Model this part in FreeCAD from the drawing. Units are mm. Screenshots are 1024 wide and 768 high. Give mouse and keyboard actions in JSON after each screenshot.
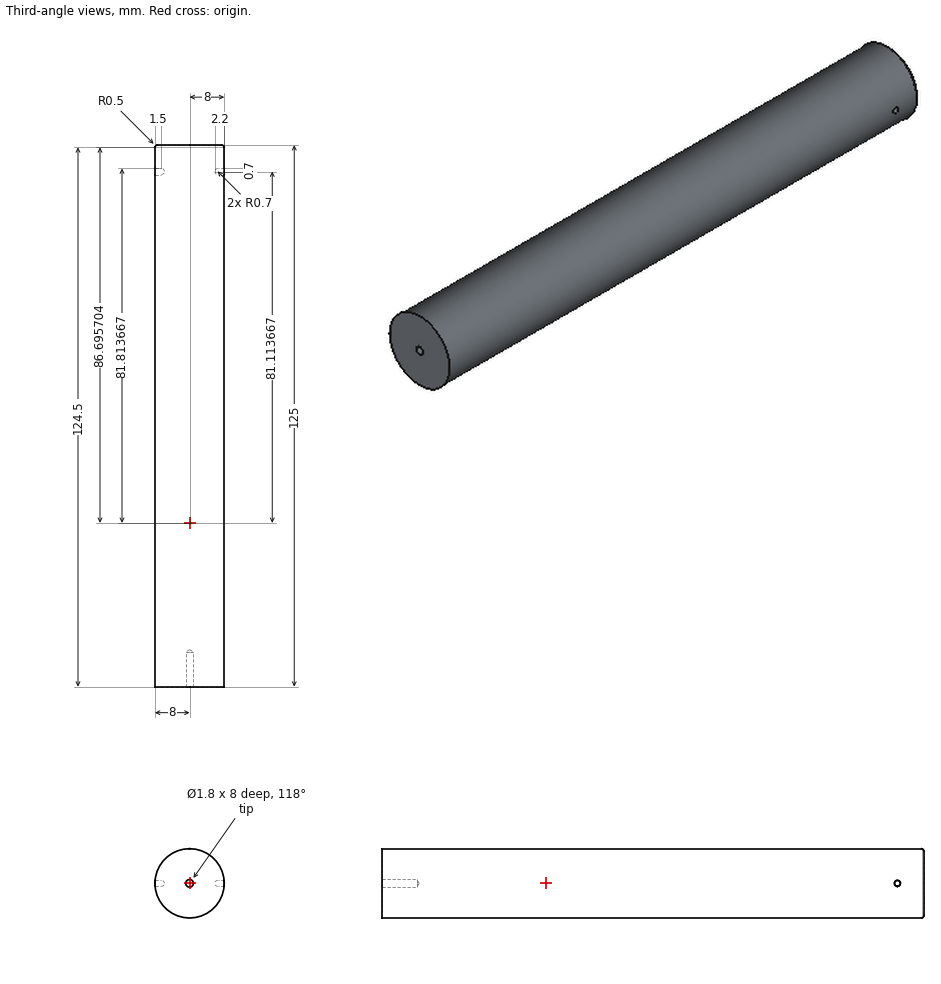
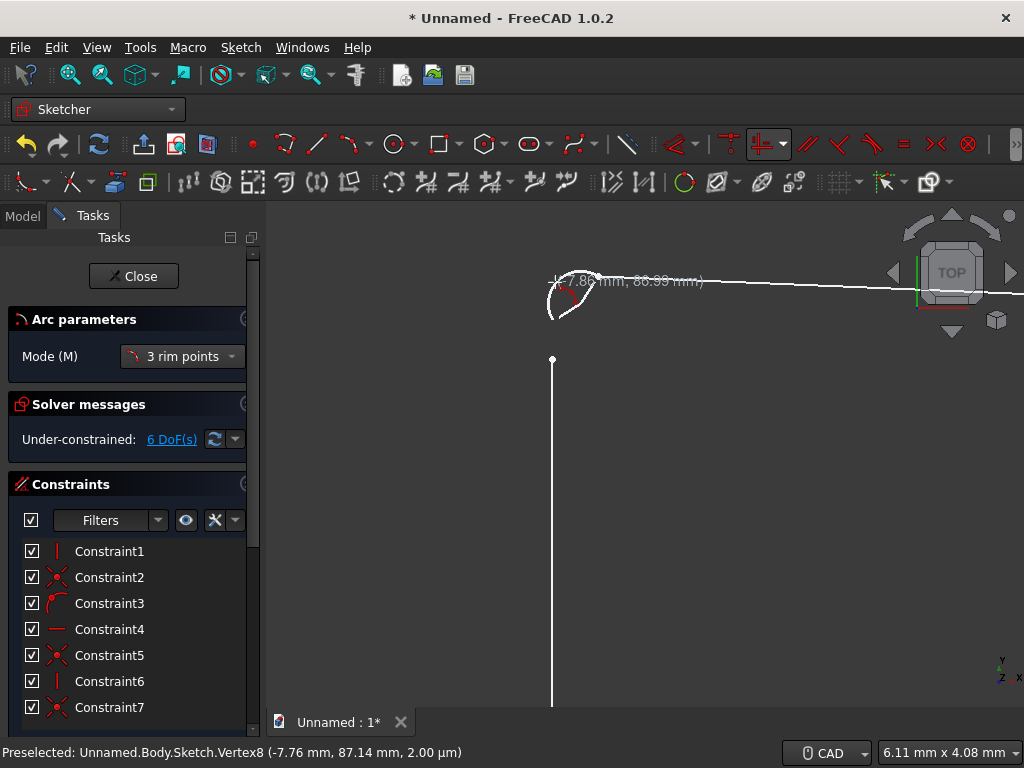
{"action": "left_click", "coordinate": [554, 279]}
{"action": "key", "text": "Escape"}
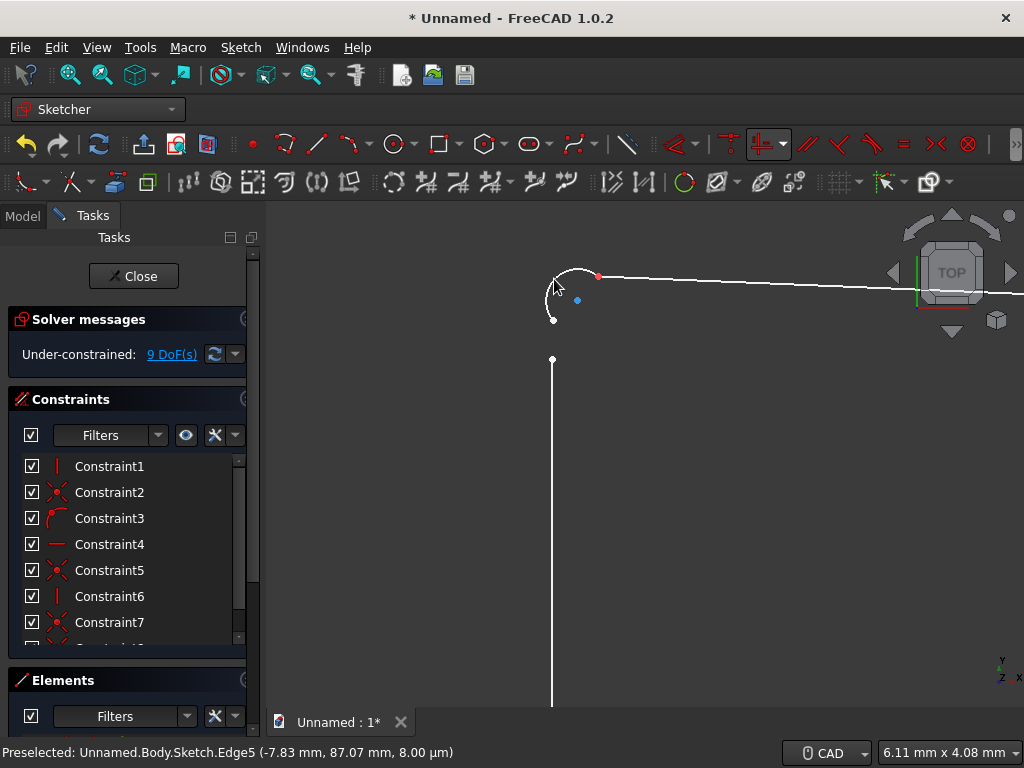
{"action": "scroll", "coordinate": [576, 454], "scroll_direction": "down", "scroll_amount": 15}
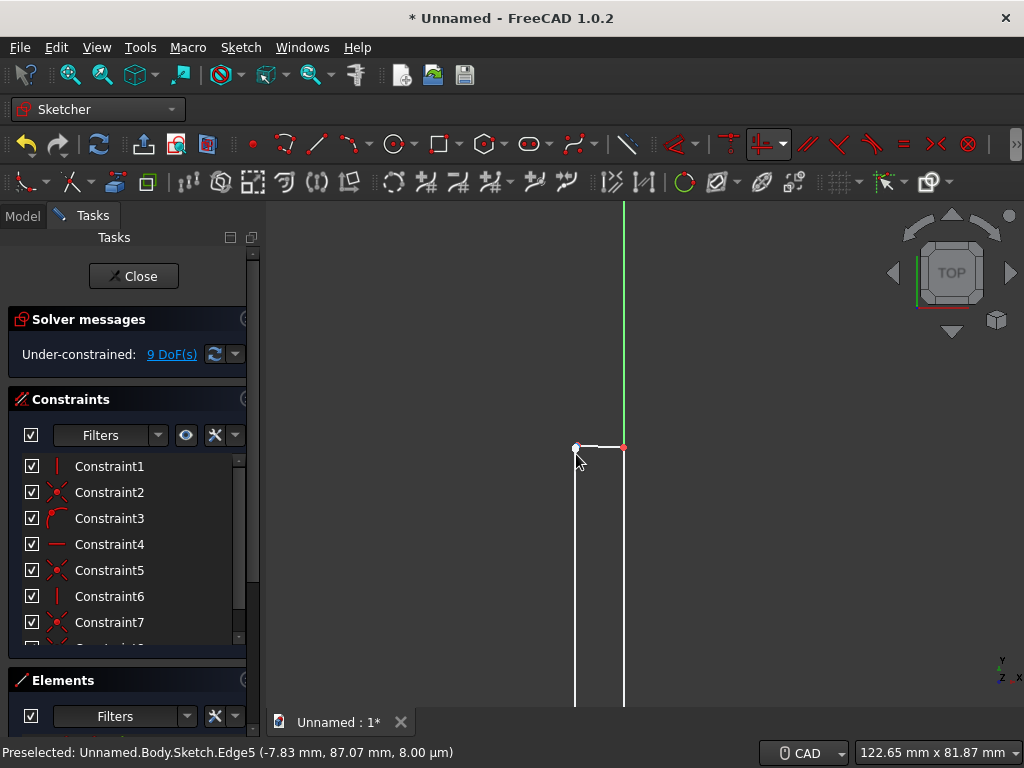
{"action": "scroll", "coordinate": [563, 235], "scroll_direction": "down", "scroll_amount": 5}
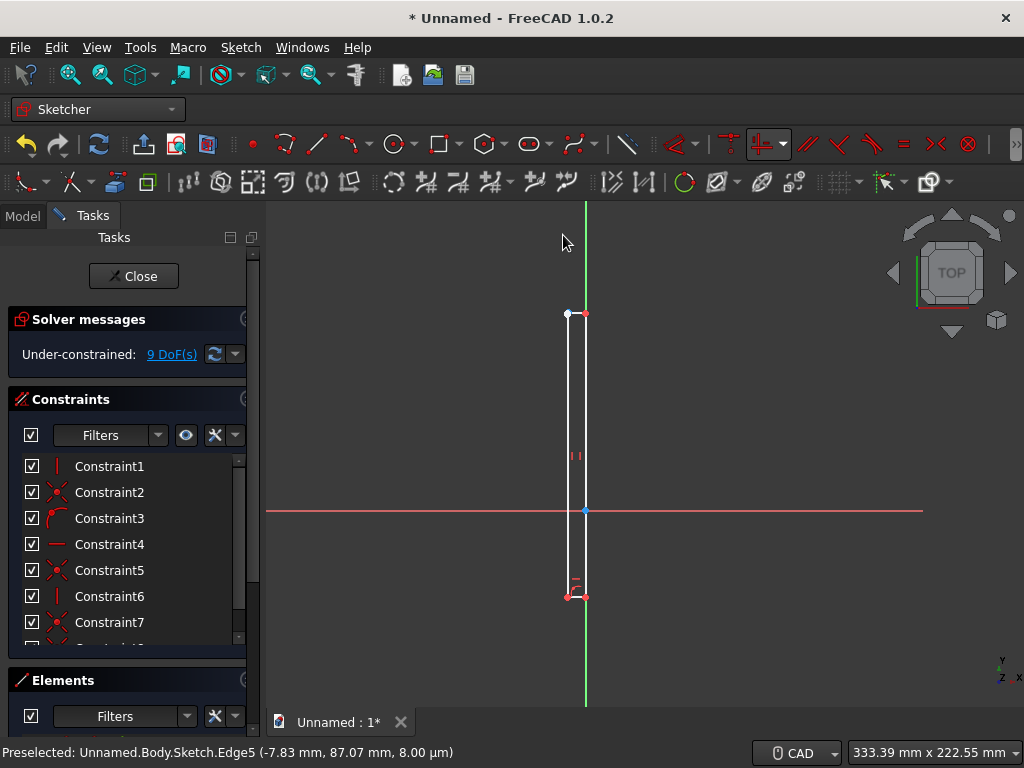
{"action": "left_click", "coordinate": [568, 399]}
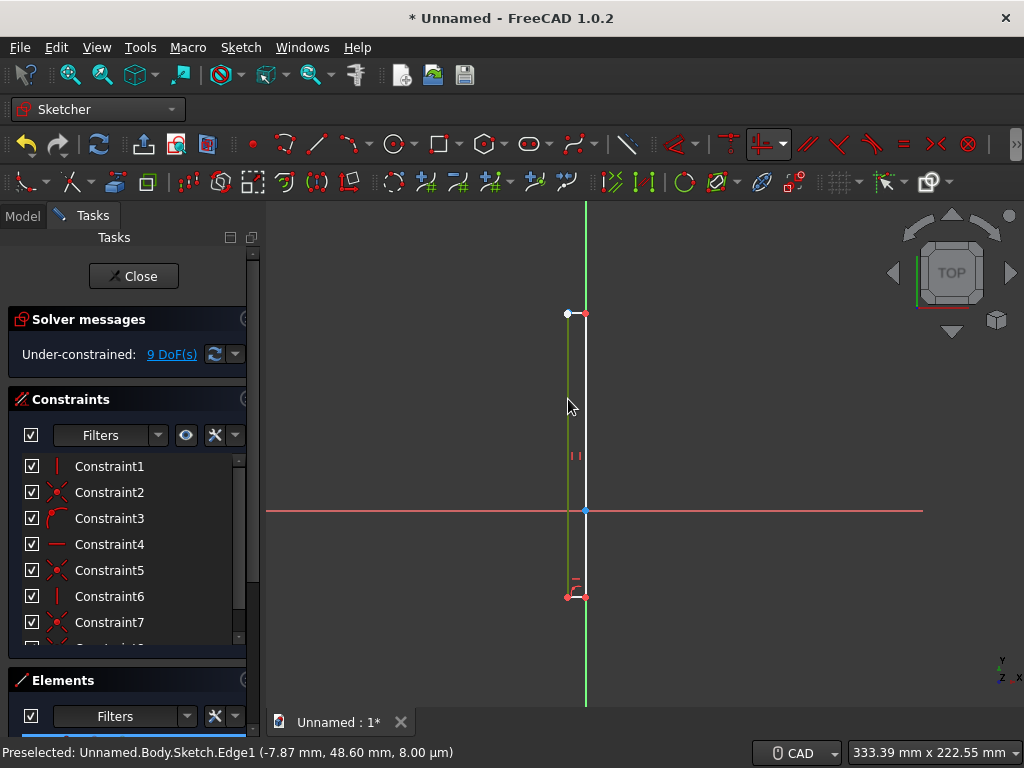
{"action": "scroll", "coordinate": [568, 313], "scroll_direction": "up", "scroll_amount": 15}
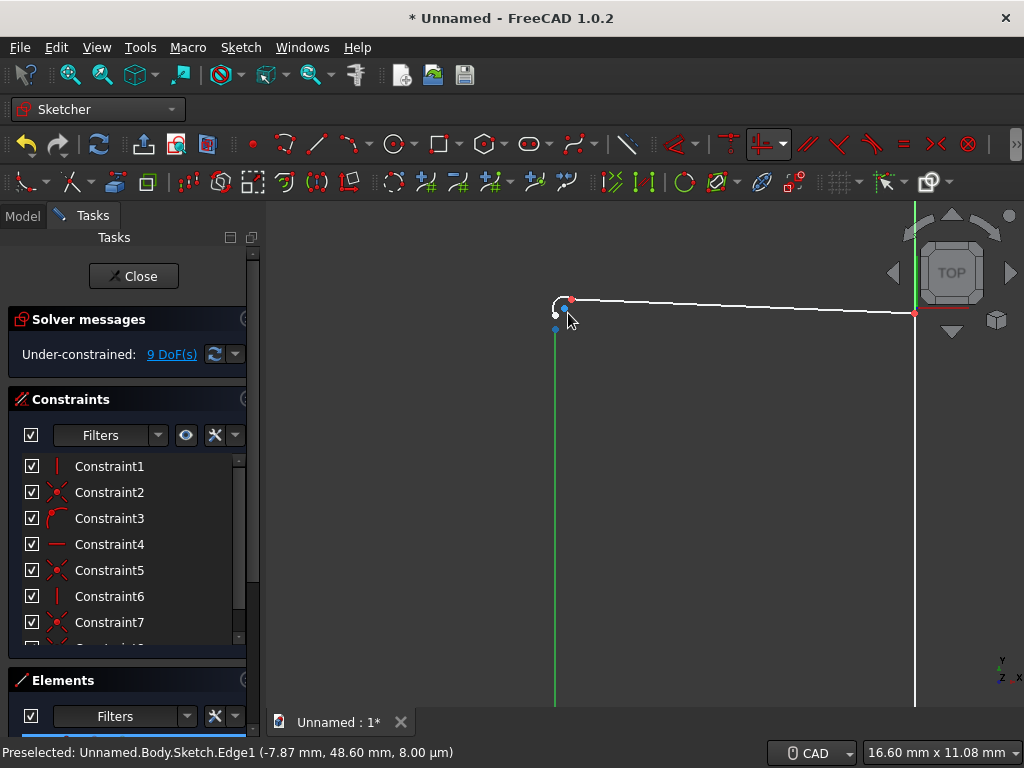
{"action": "left_click", "coordinate": [556, 300]}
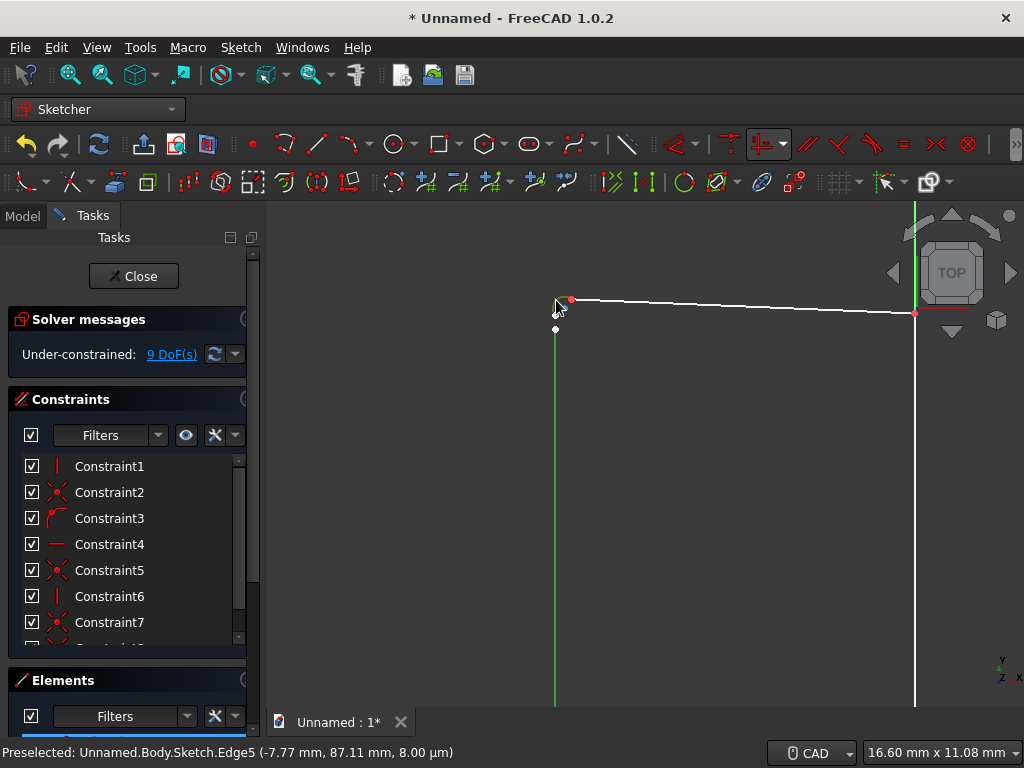
{"action": "key", "text": "t"}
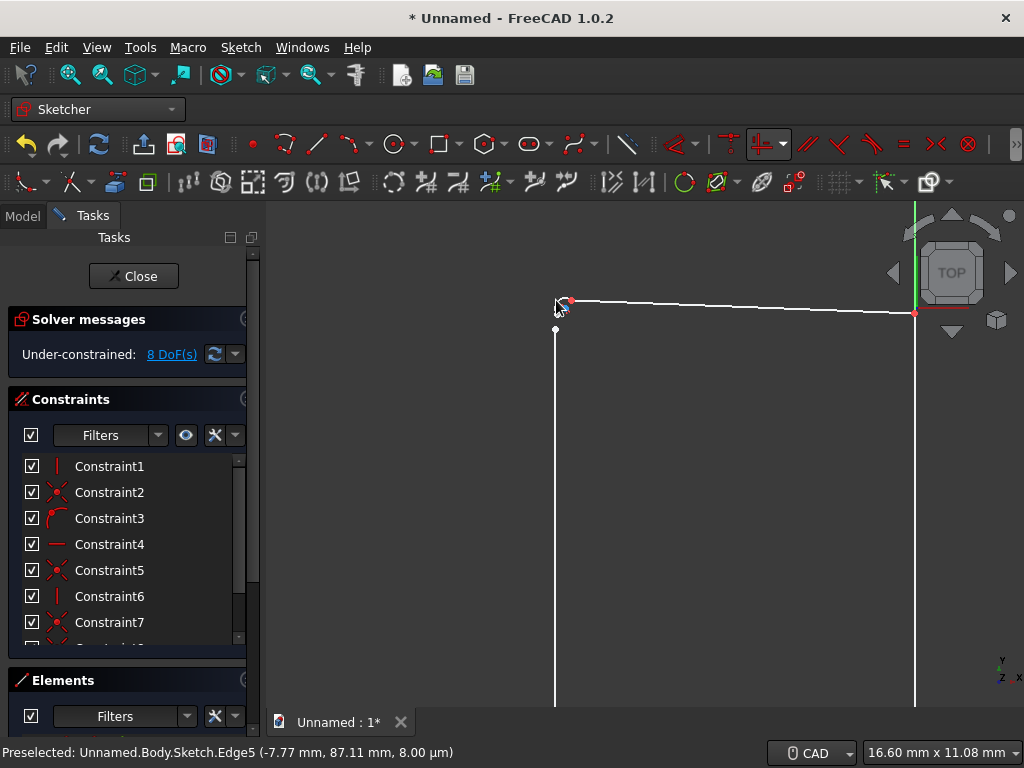
{"action": "scroll", "coordinate": [566, 280], "scroll_direction": "down", "scroll_amount": 14}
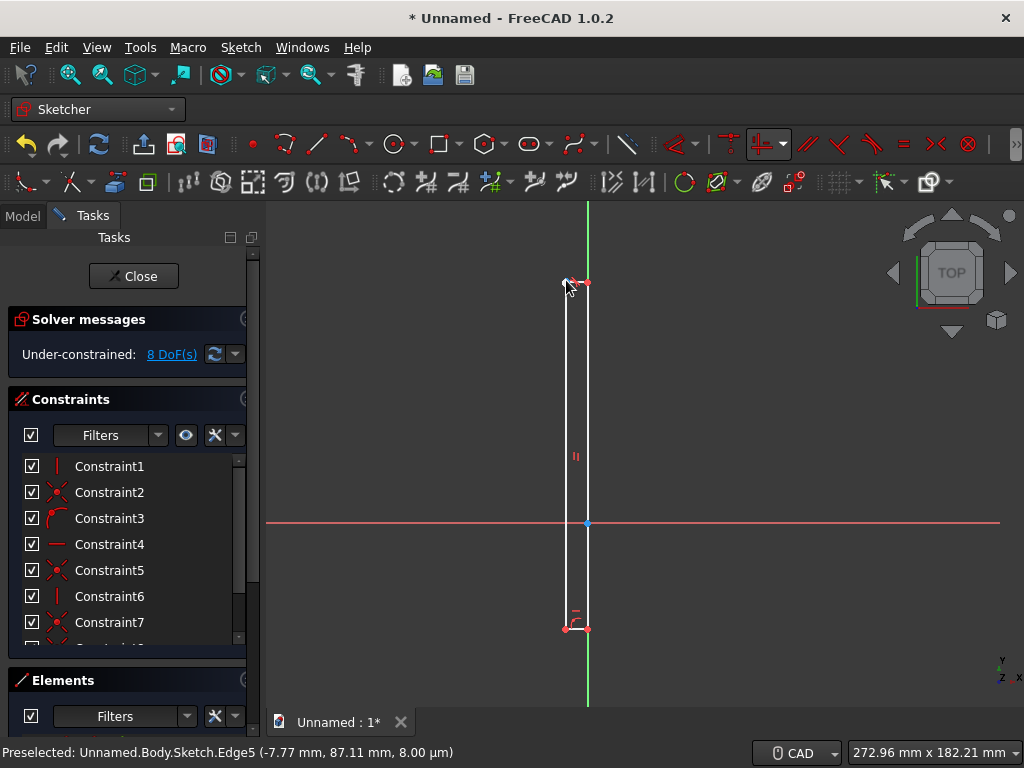
{"action": "scroll", "coordinate": [581, 282], "scroll_direction": "up", "scroll_amount": 4}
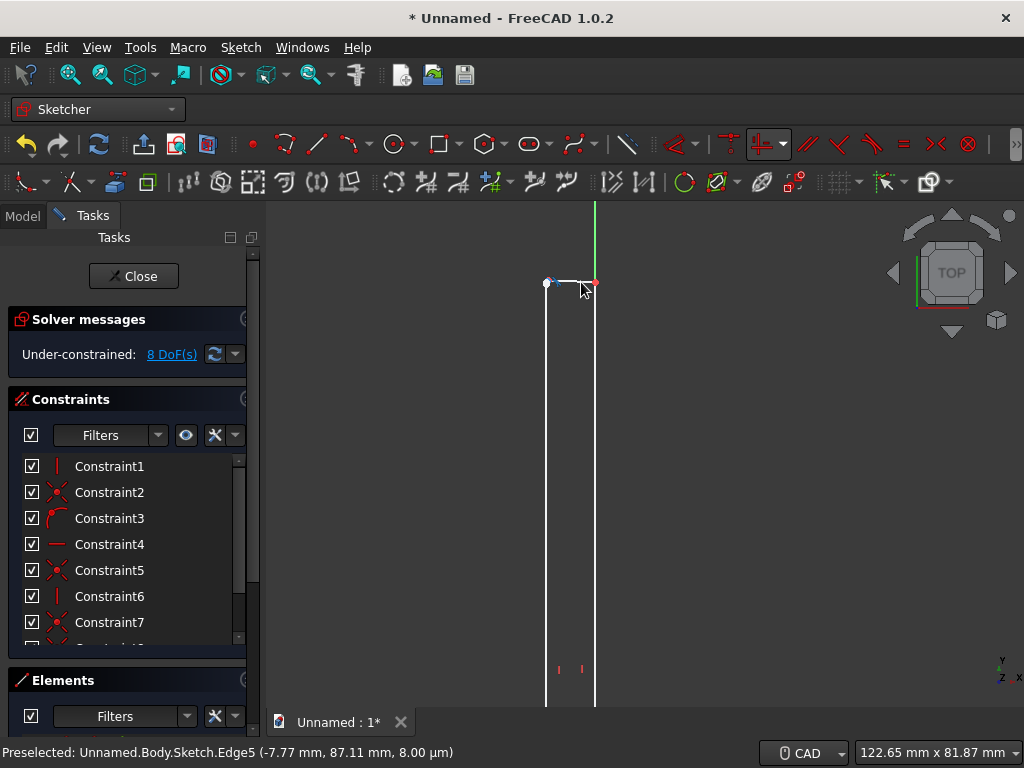
{"action": "left_click", "coordinate": [581, 282]}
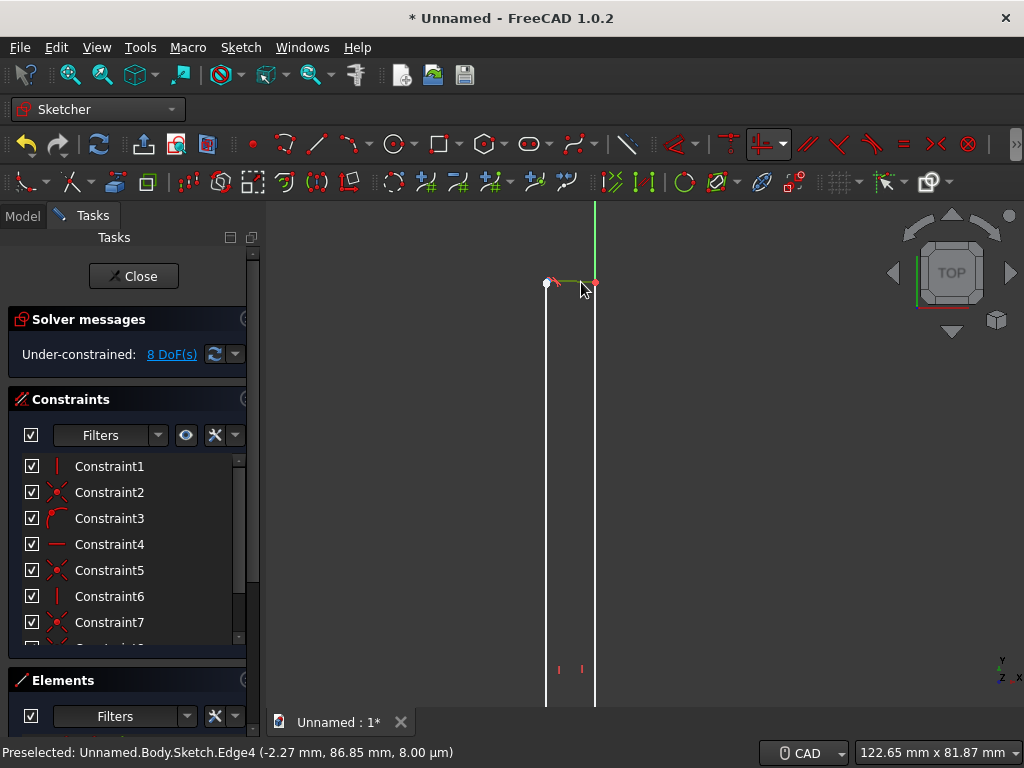
{"action": "scroll", "coordinate": [547, 281], "scroll_direction": "up", "scroll_amount": 10}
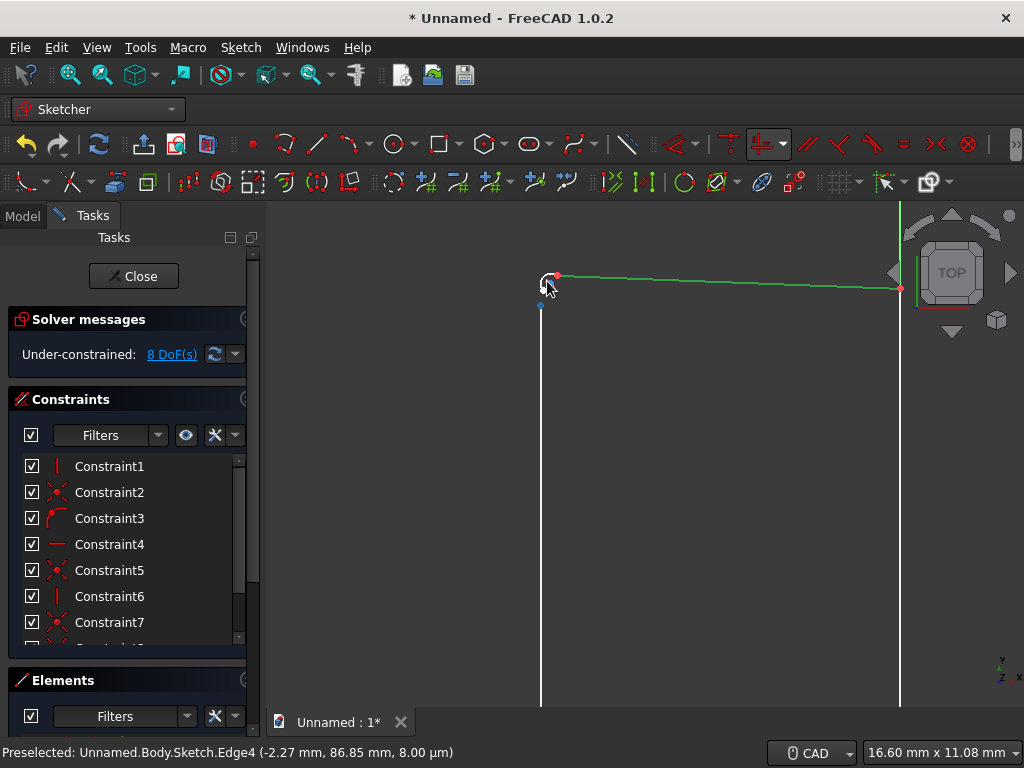
{"action": "left_click", "coordinate": [544, 277]}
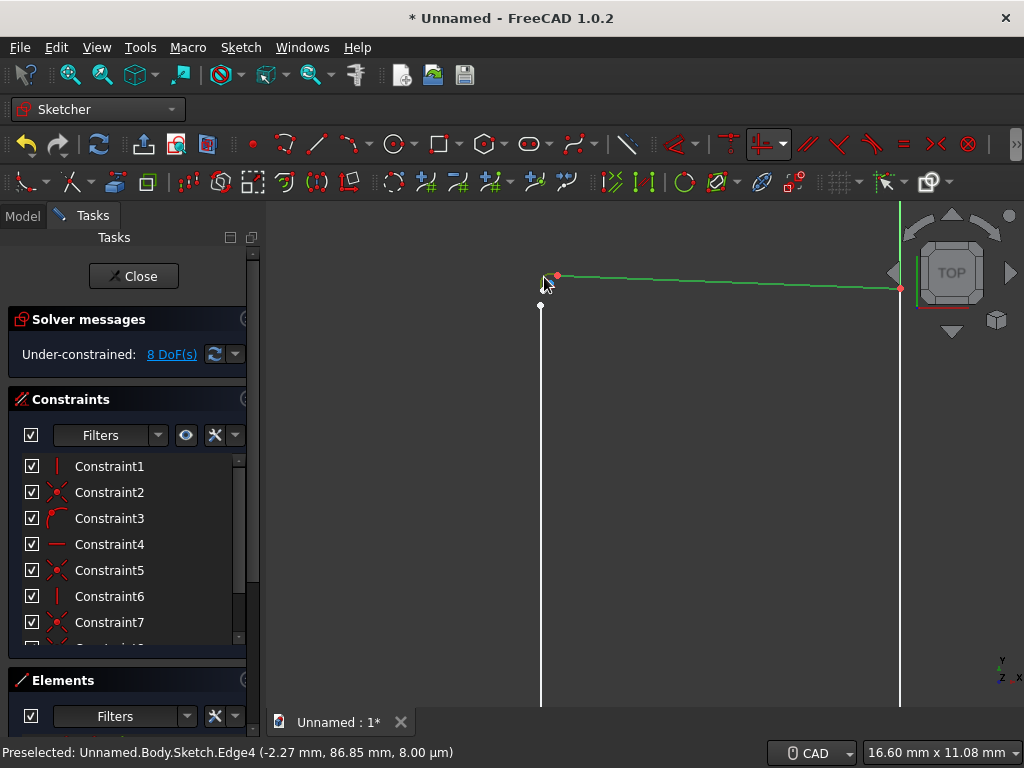
{"action": "key", "text": "t"}